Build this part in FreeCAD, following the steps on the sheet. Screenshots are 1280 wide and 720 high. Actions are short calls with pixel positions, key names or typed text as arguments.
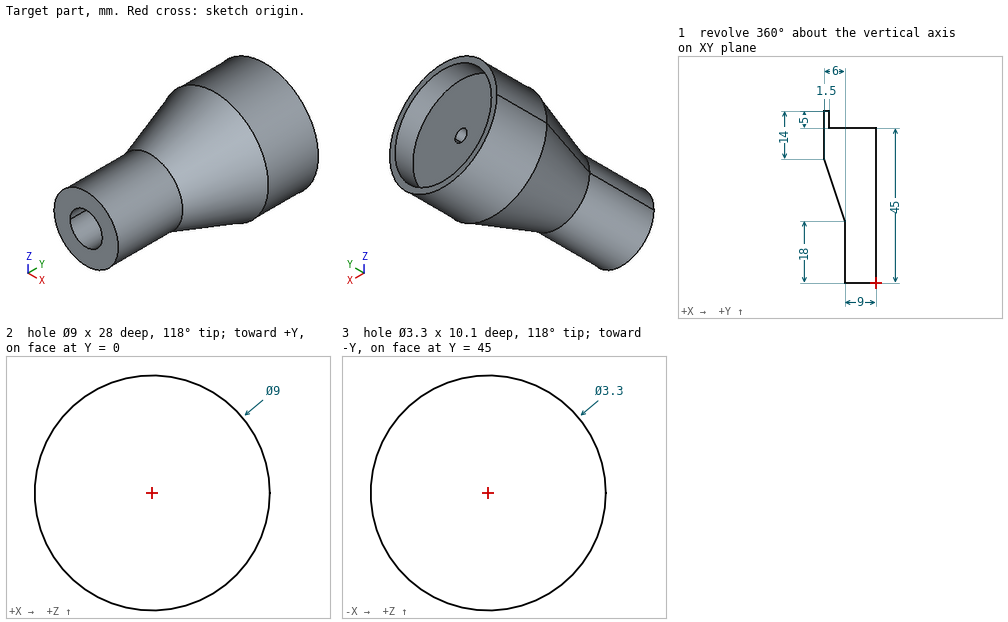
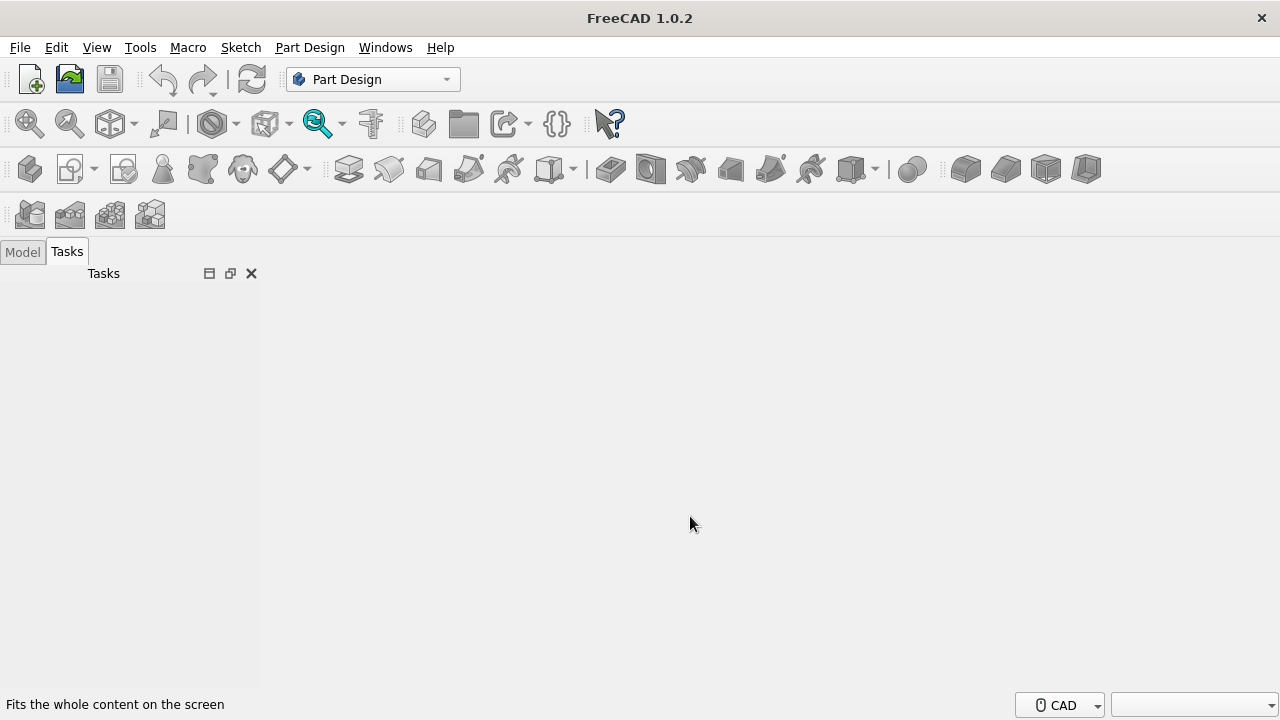
click(30, 80)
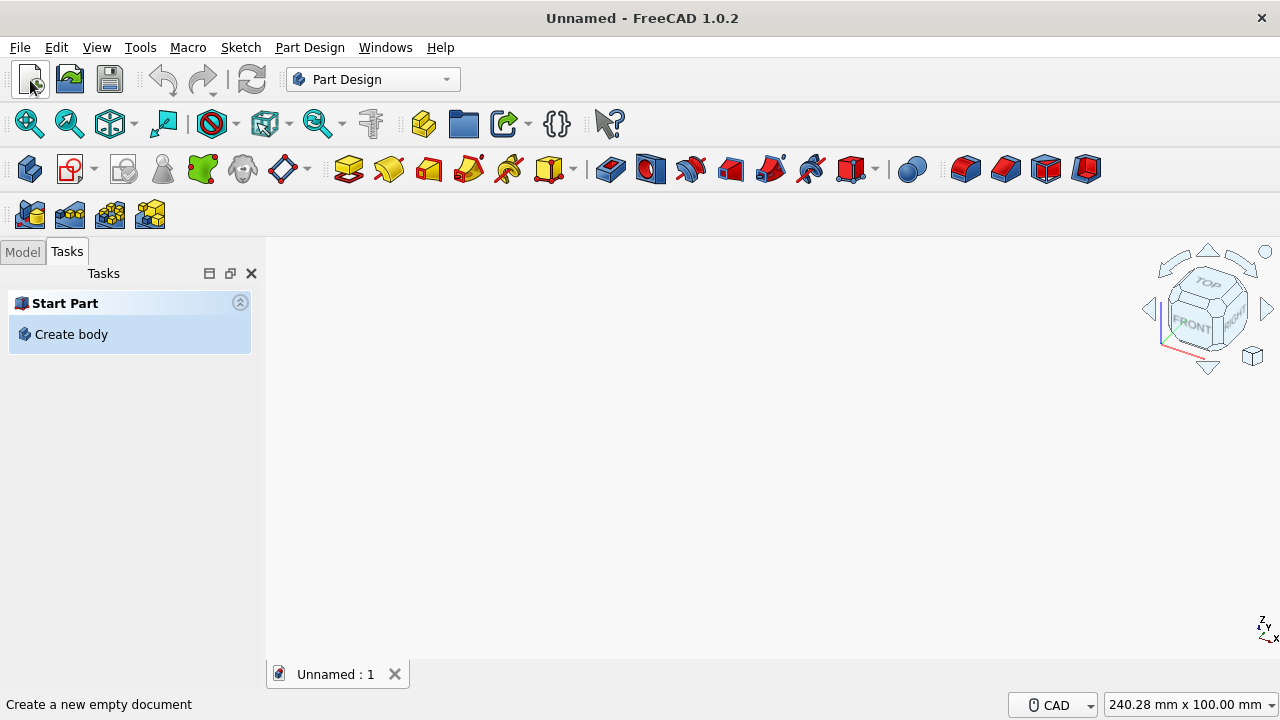
click(70, 170)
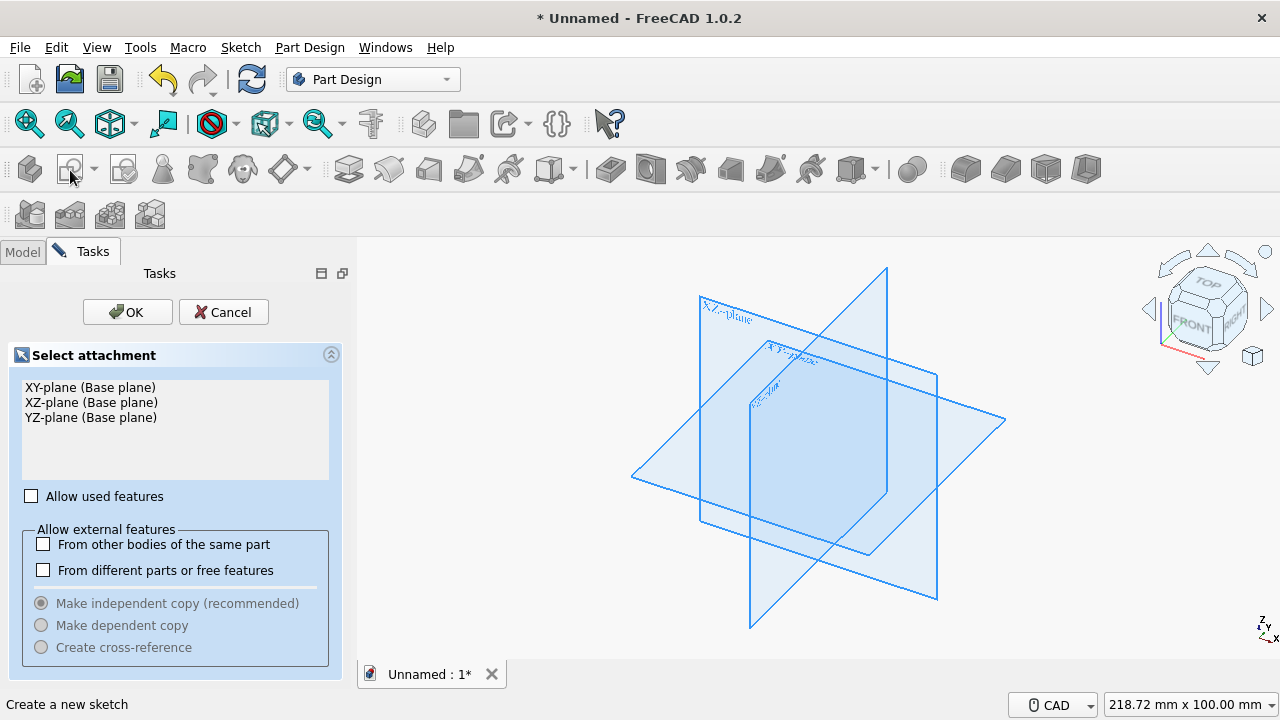
click(82, 388)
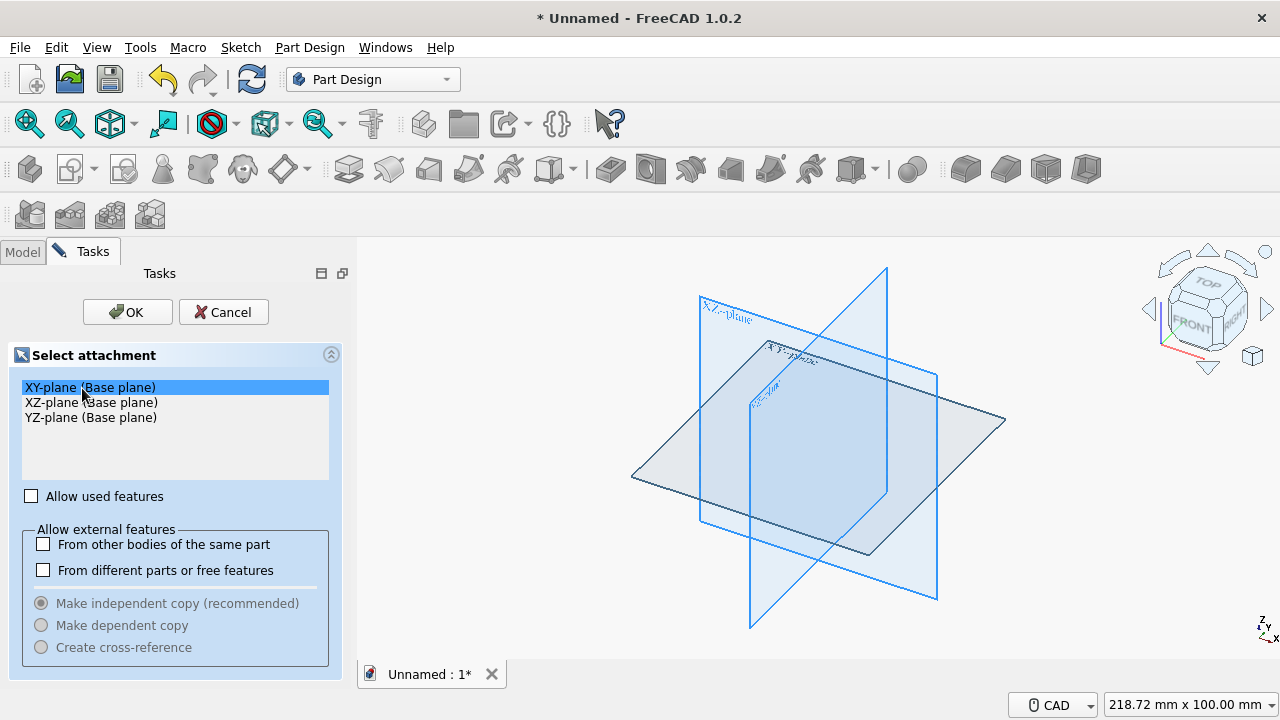
click(128, 312)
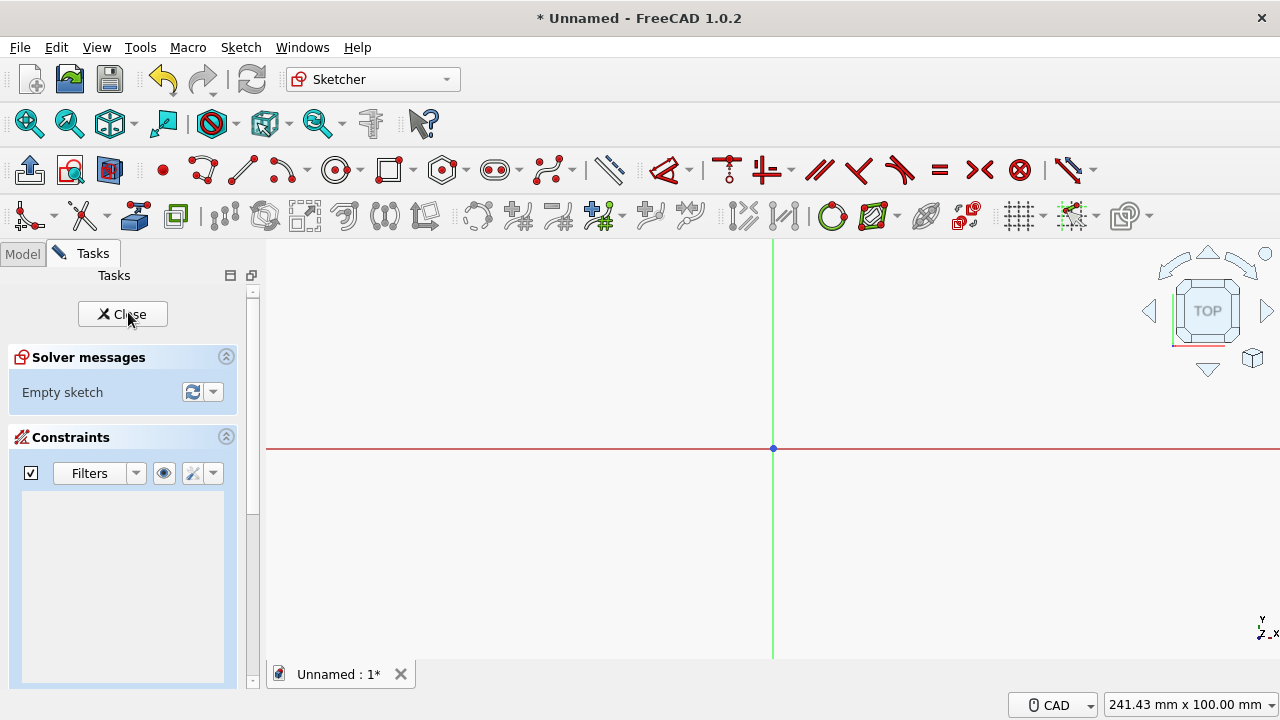
scroll(537, 631, down, 1)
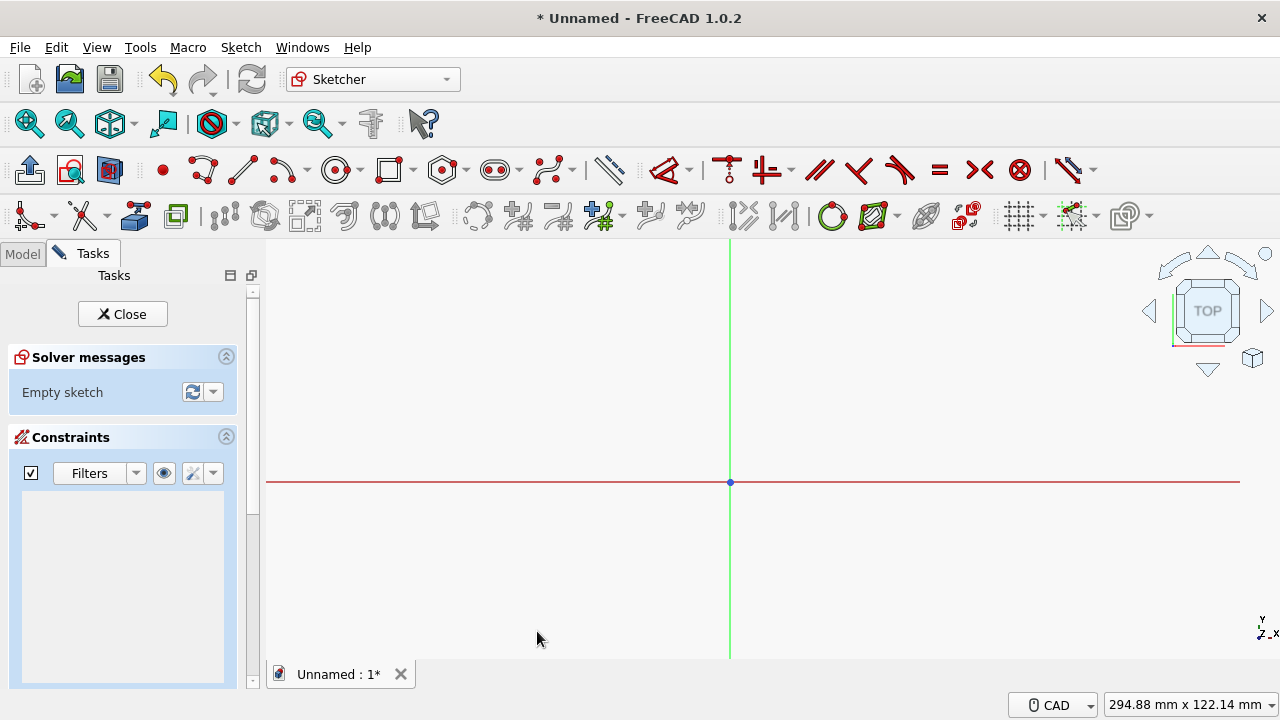
scroll(704, 289, up, 2)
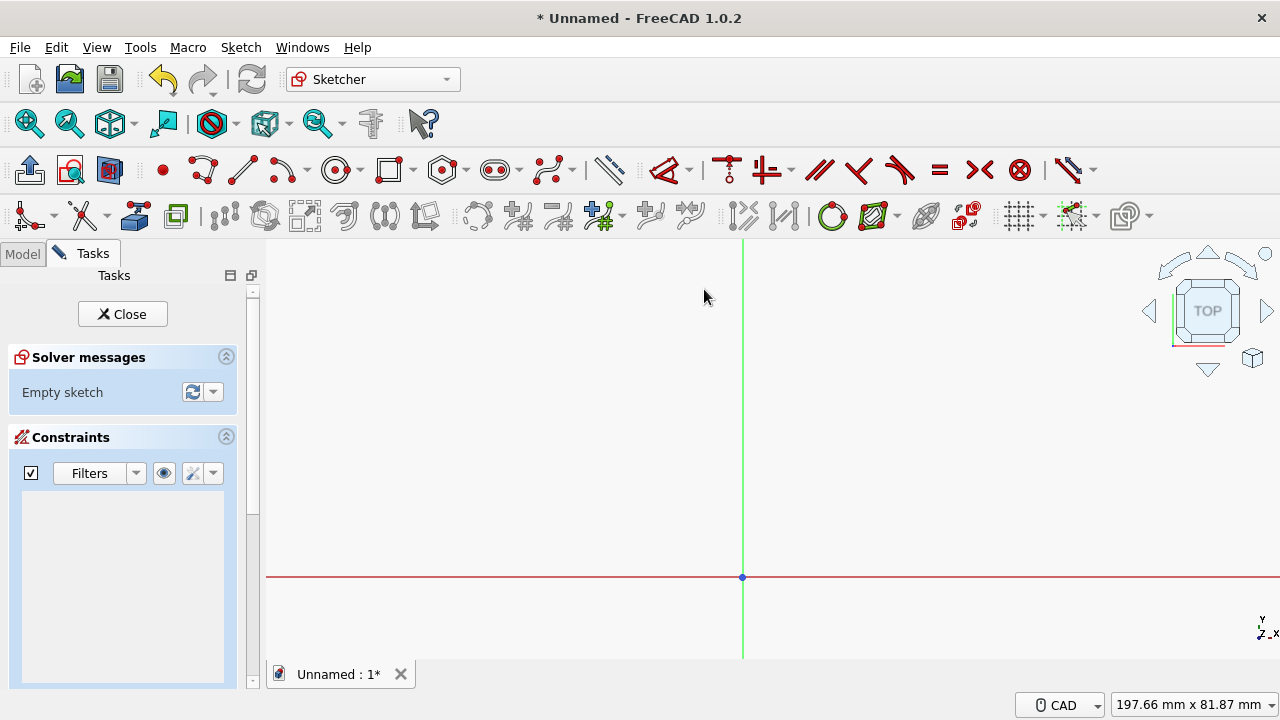
click(204, 170)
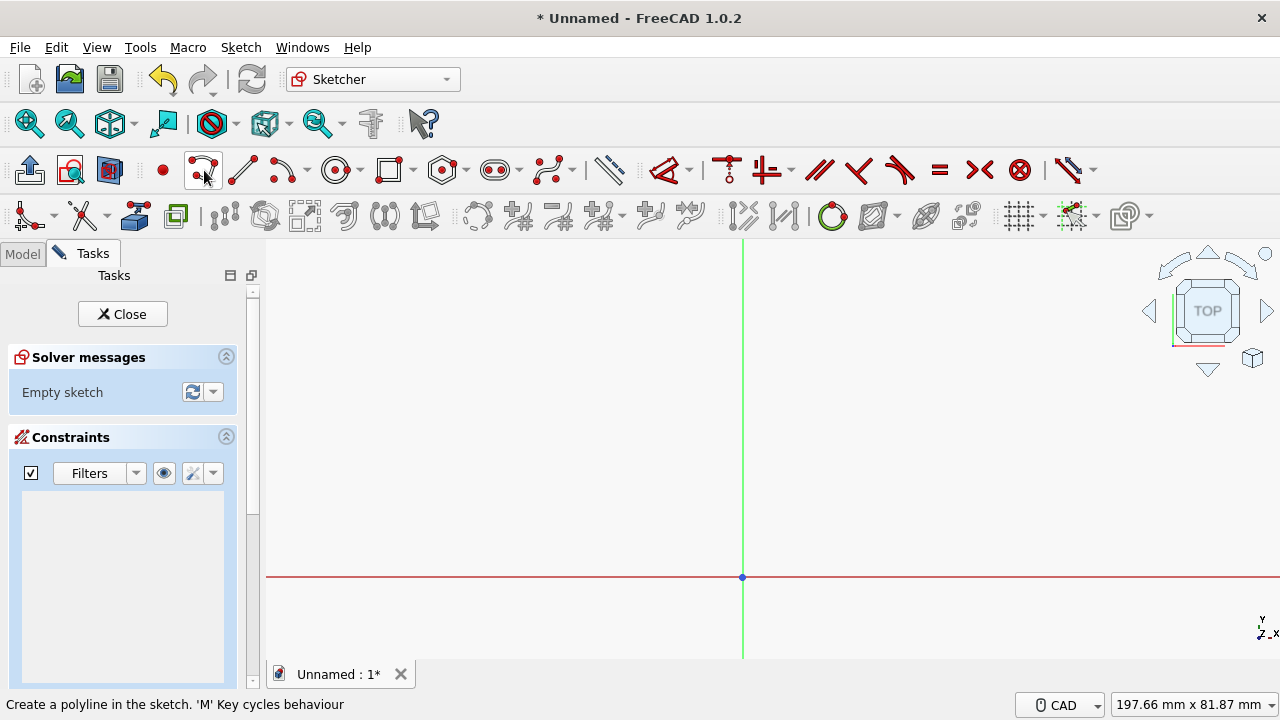
click(743, 577)
click(734, 346)
click(674, 346)
click(674, 321)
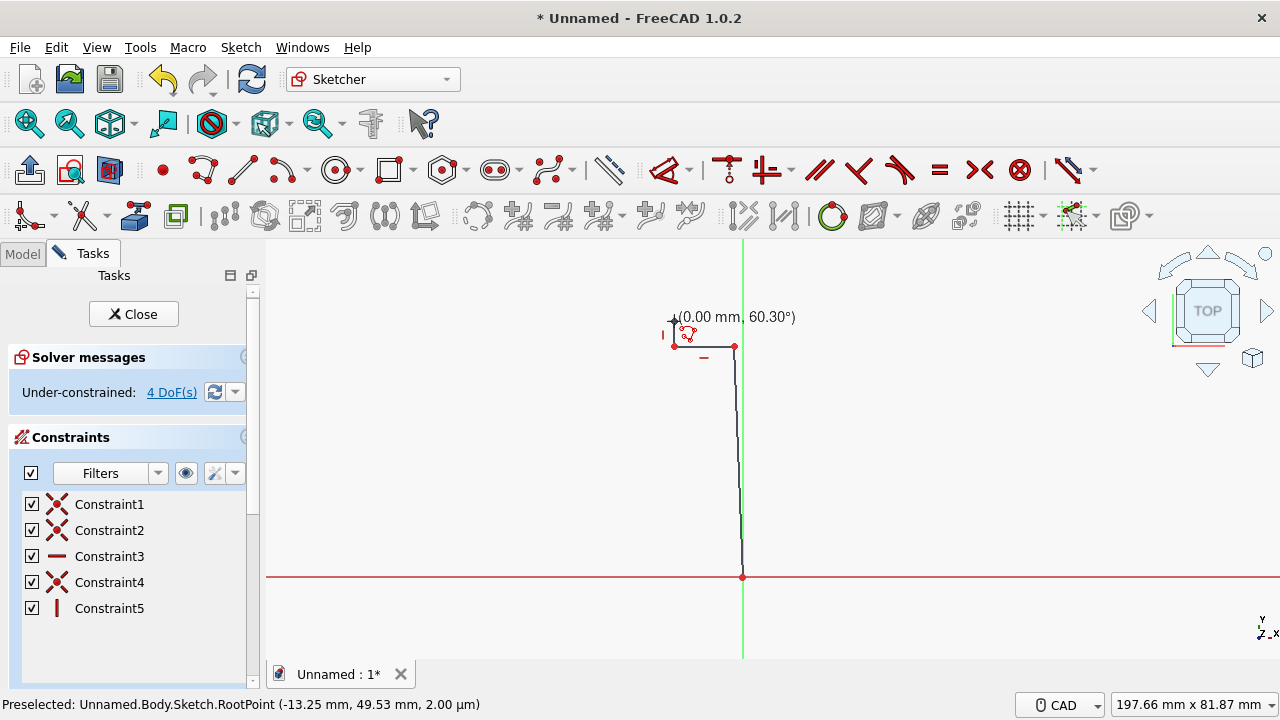
scroll(666, 321, up, 4)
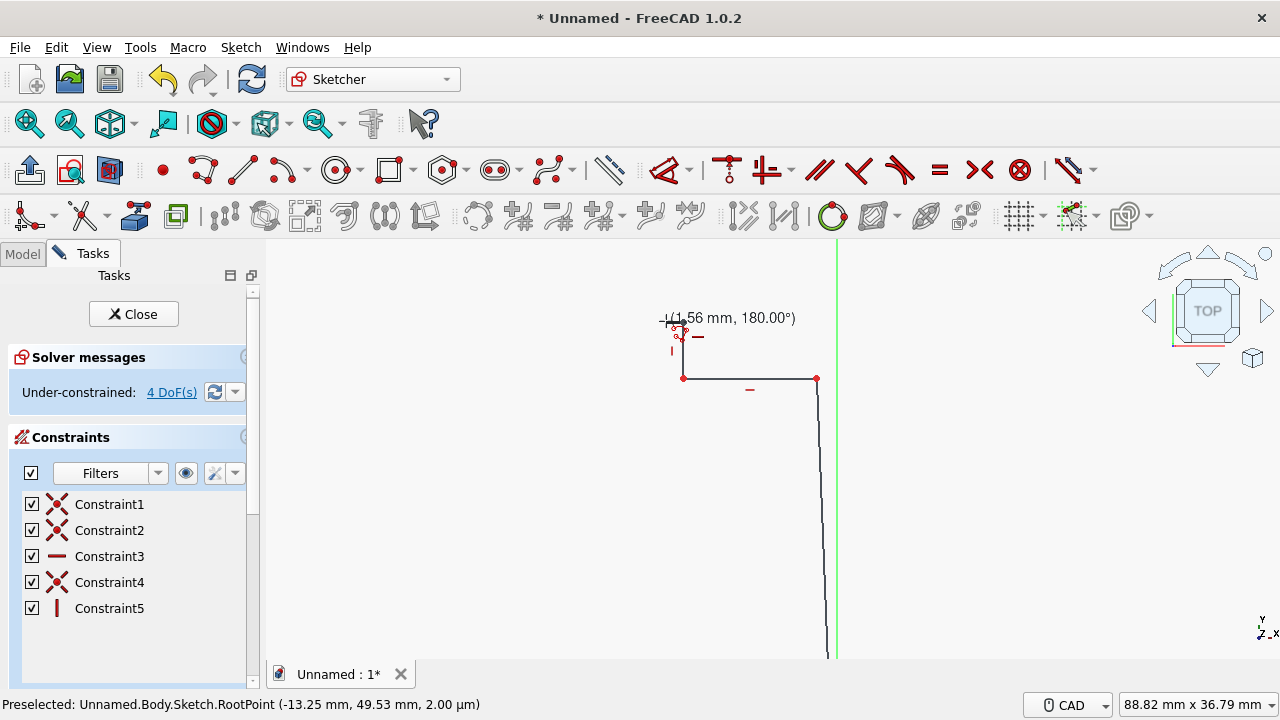
click(666, 321)
click(666, 480)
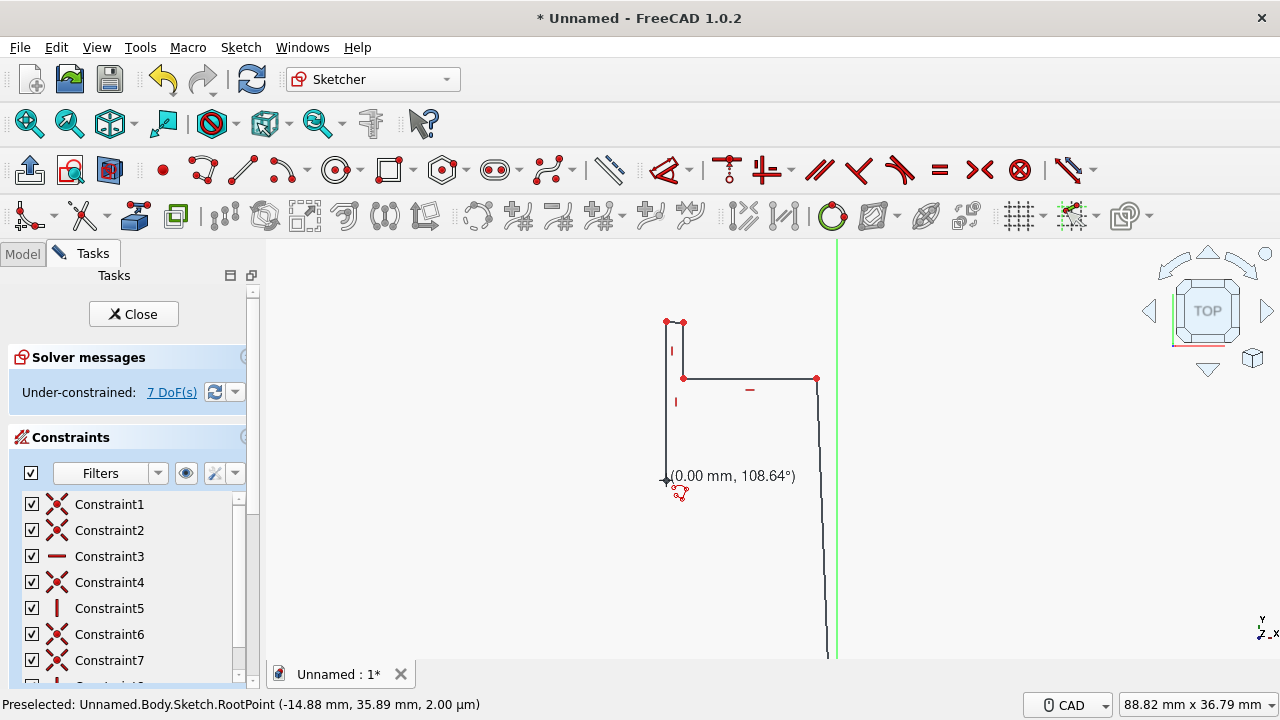
scroll(666, 321, down, 4)